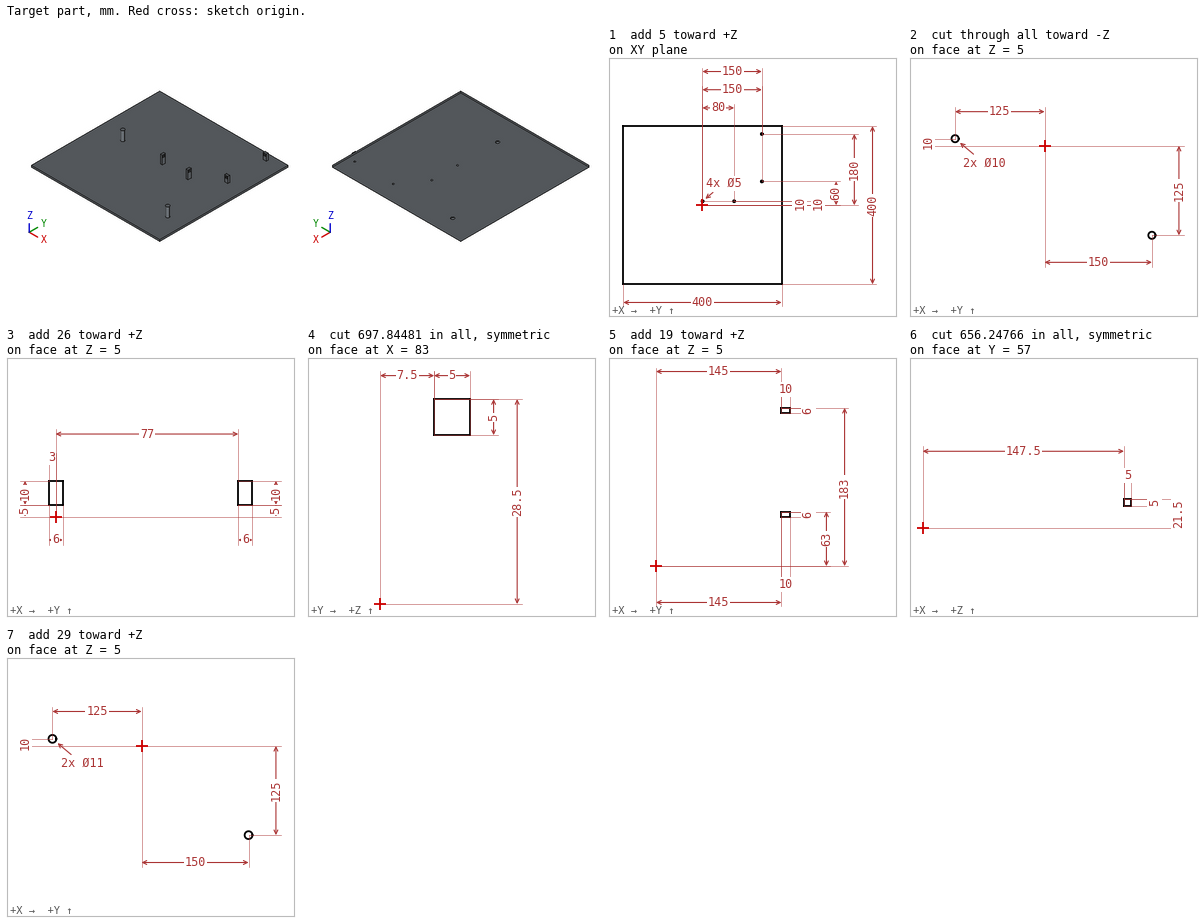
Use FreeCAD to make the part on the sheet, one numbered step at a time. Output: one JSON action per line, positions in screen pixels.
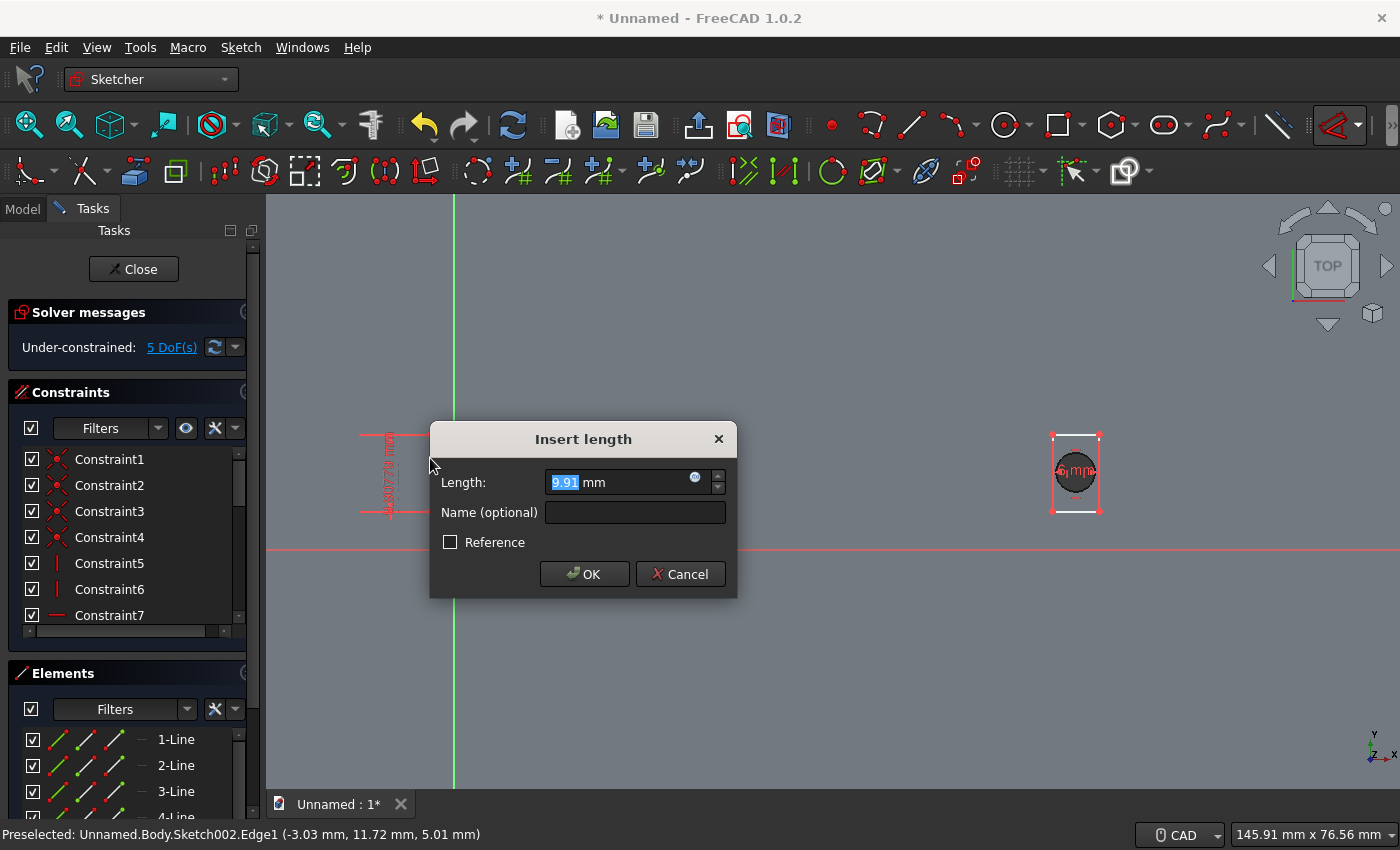
{"action": "type", "text": "10"}
{"action": "key", "text": "Return"}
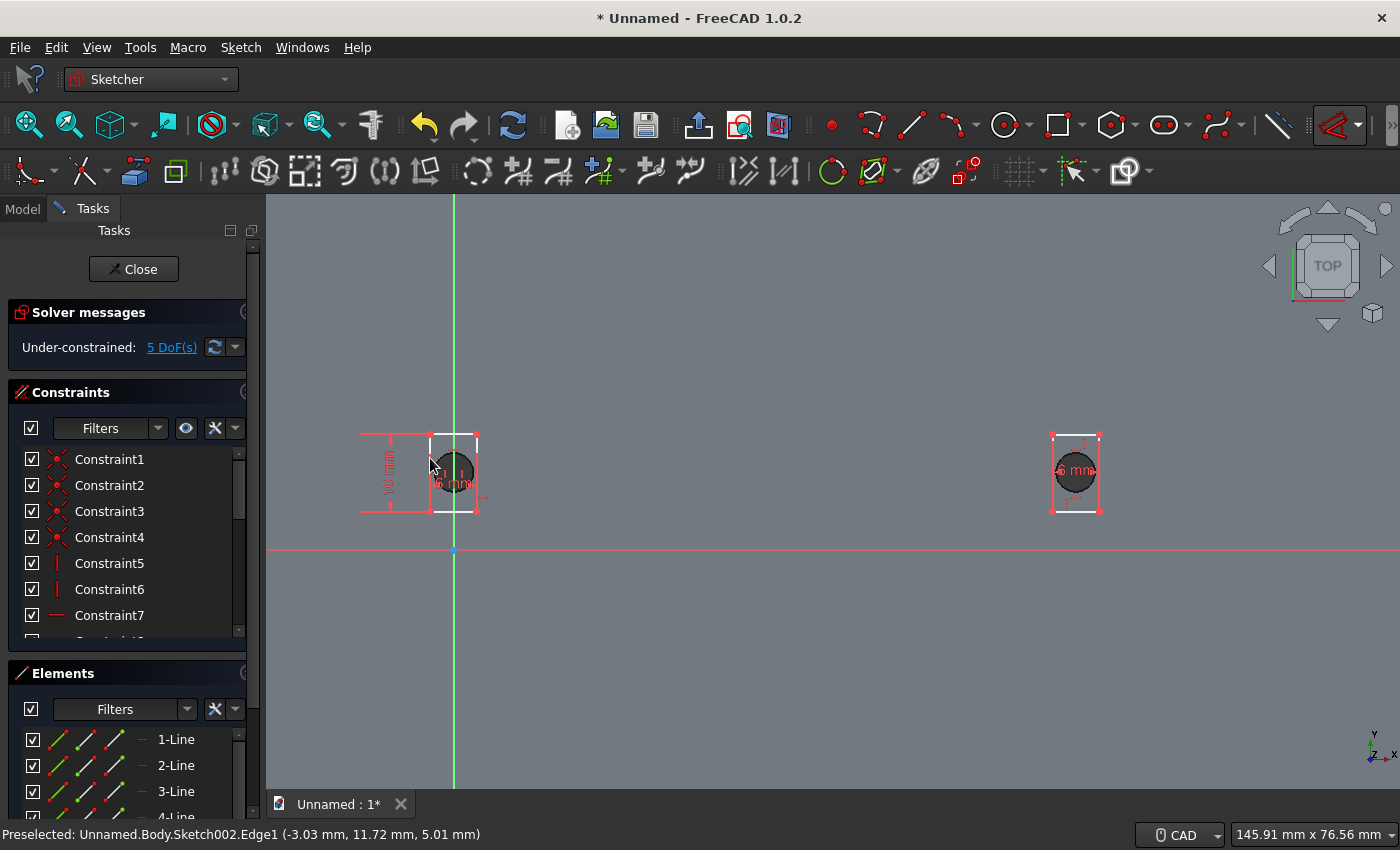
{"action": "left_click", "coordinate": [1053, 458]}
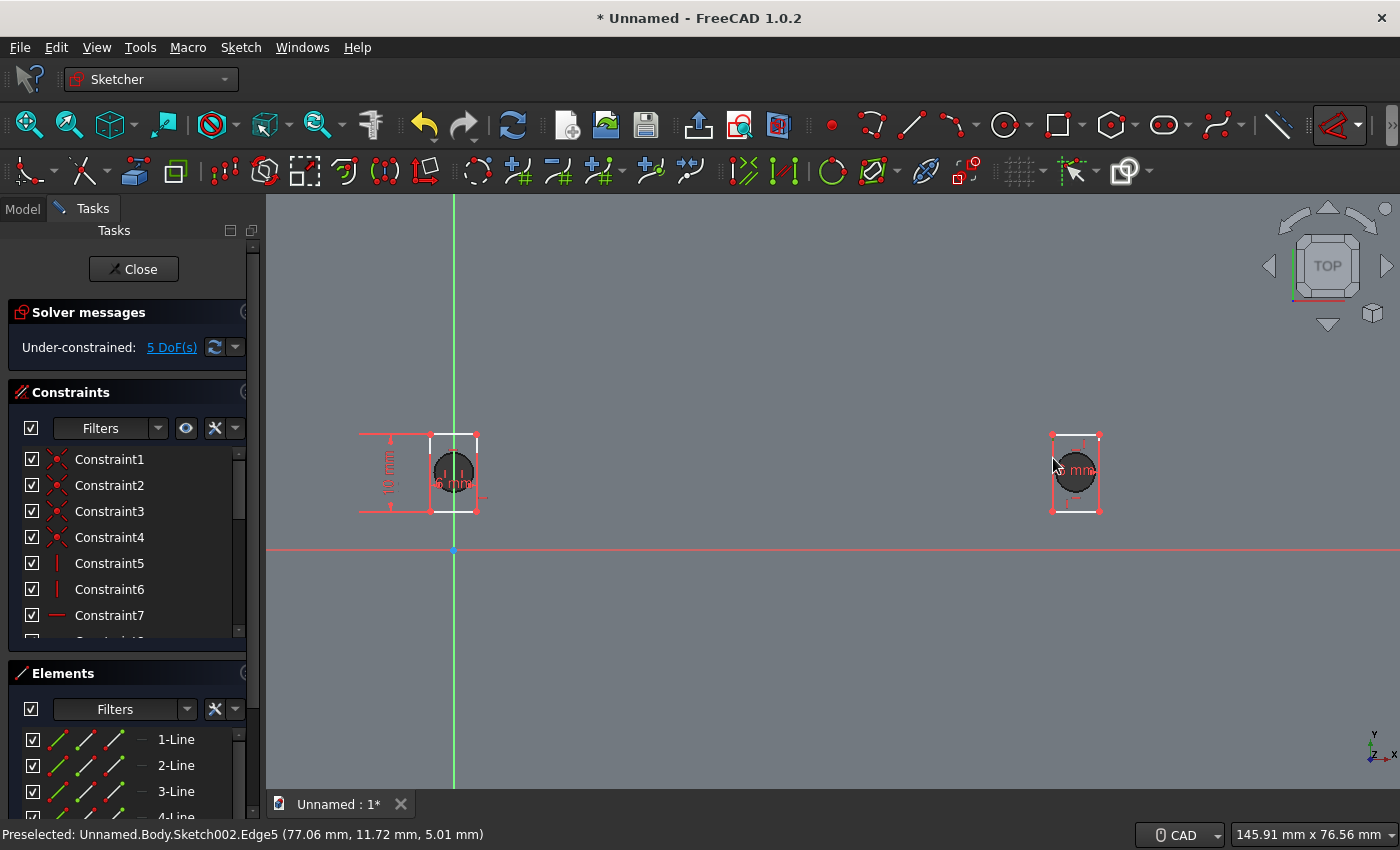
{"action": "key", "text": "i"}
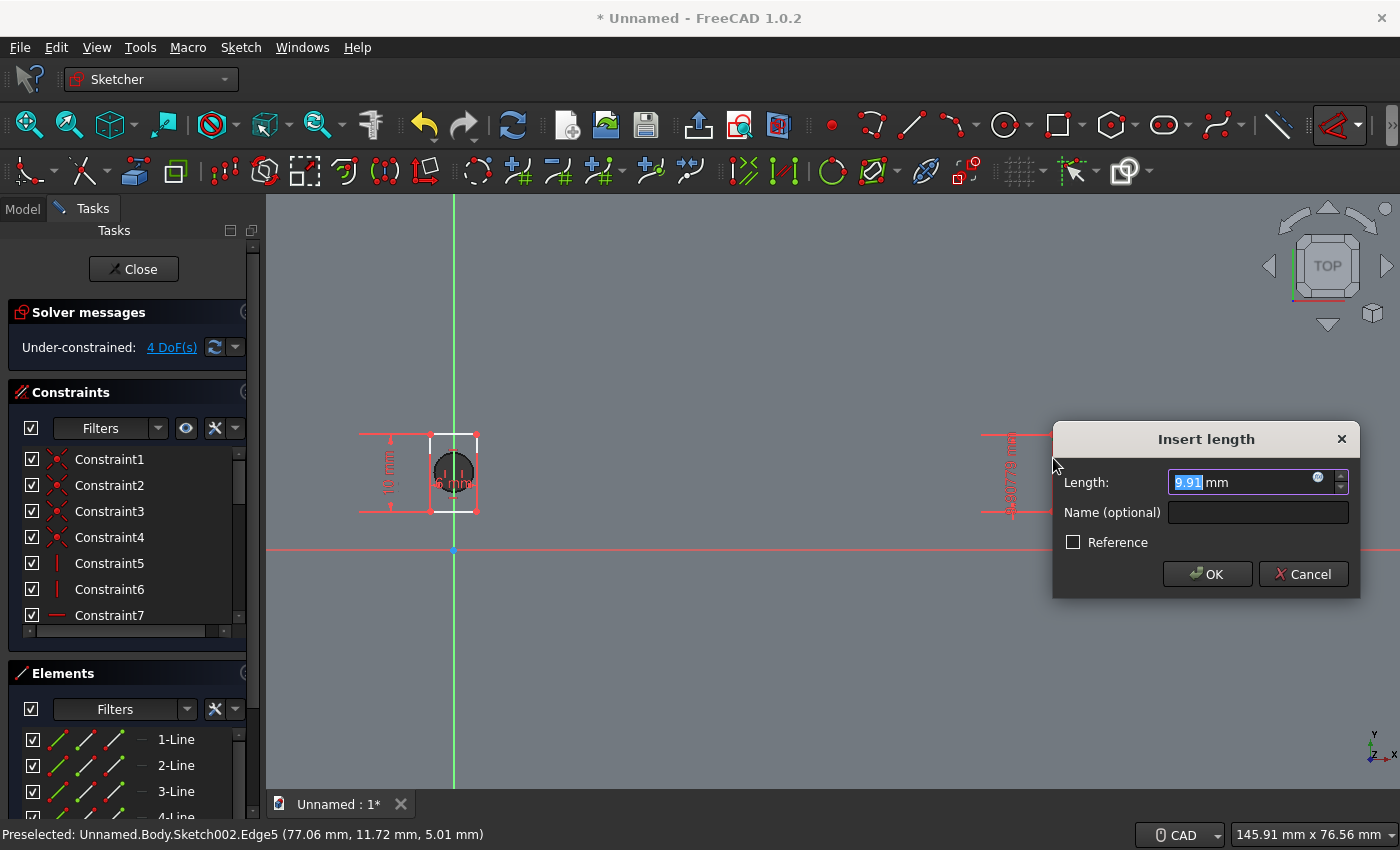
{"action": "type", "text": "10"}
{"action": "key", "text": "Return"}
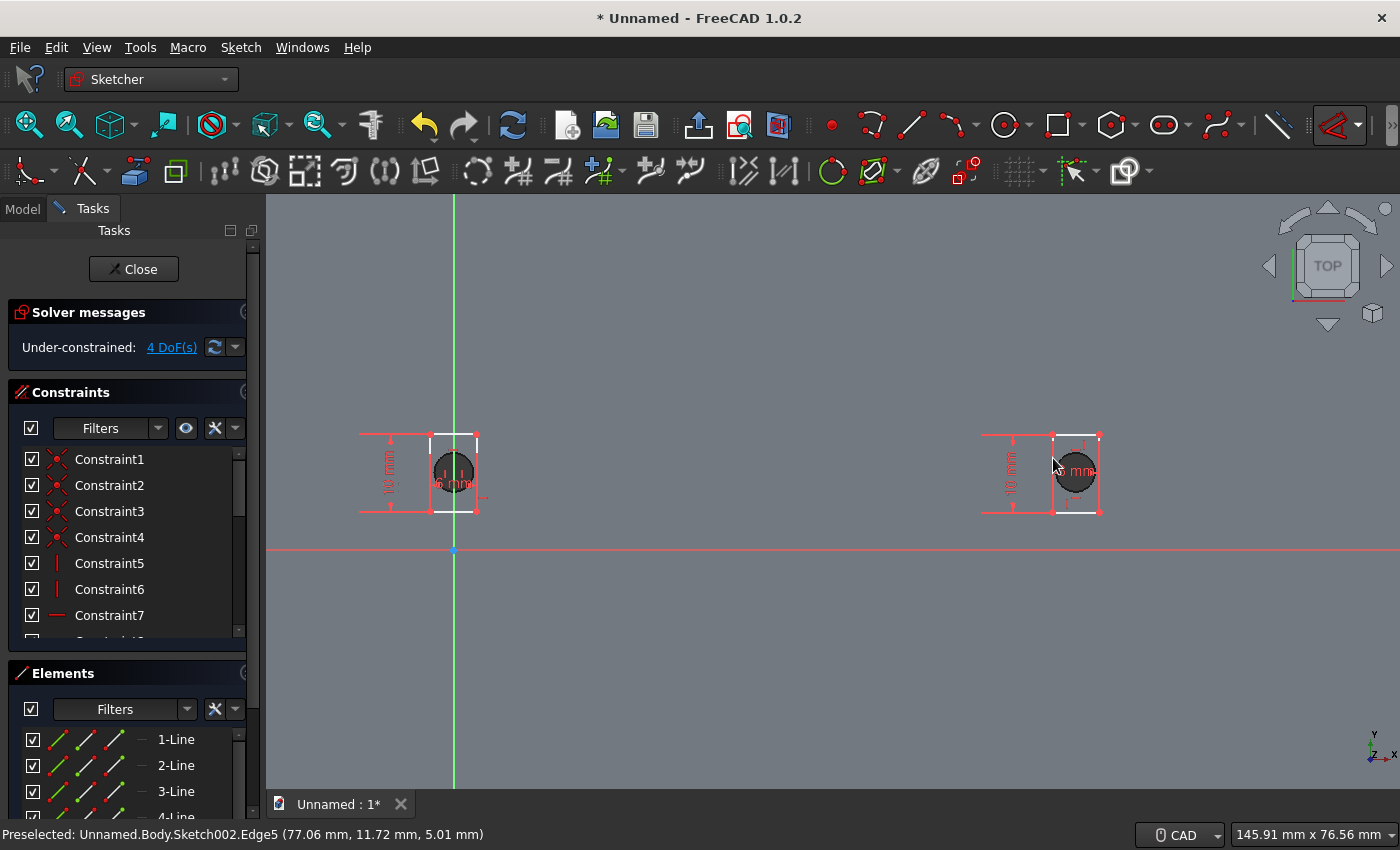
{"action": "scroll", "coordinate": [430, 434], "scroll_direction": "up", "scroll_amount": 3}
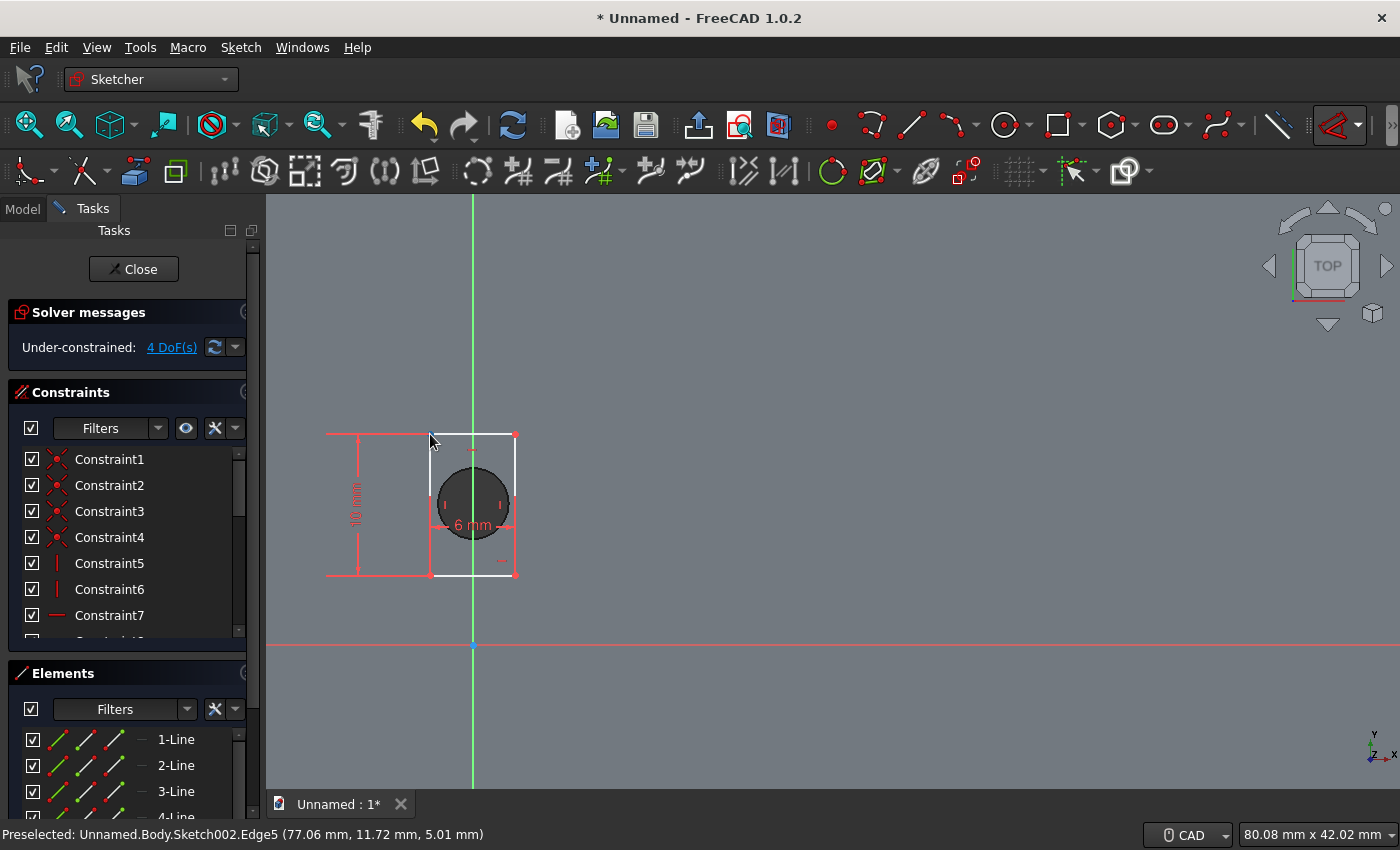
{"action": "left_click", "coordinate": [430, 434]}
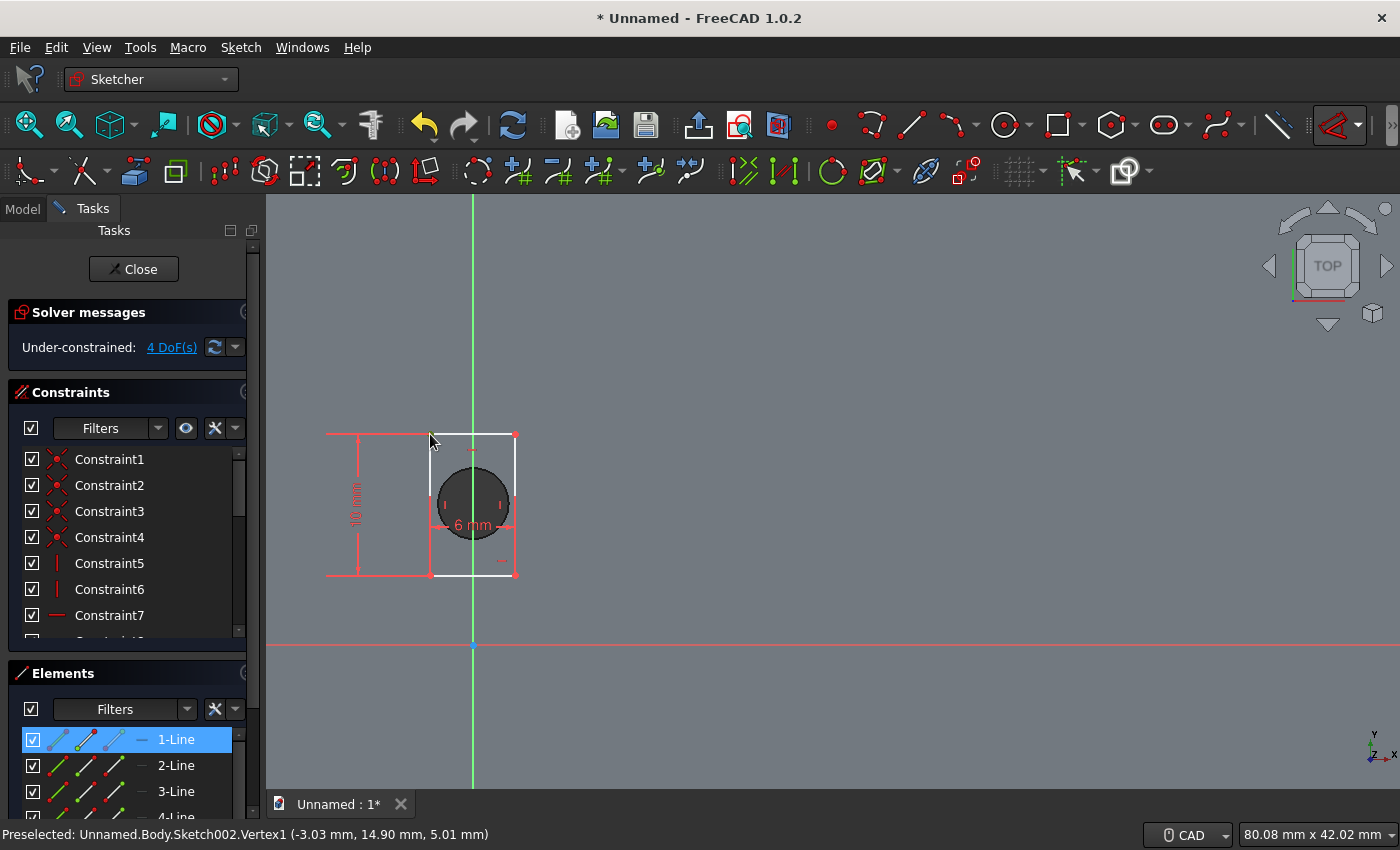
{"action": "key", "text": "l"}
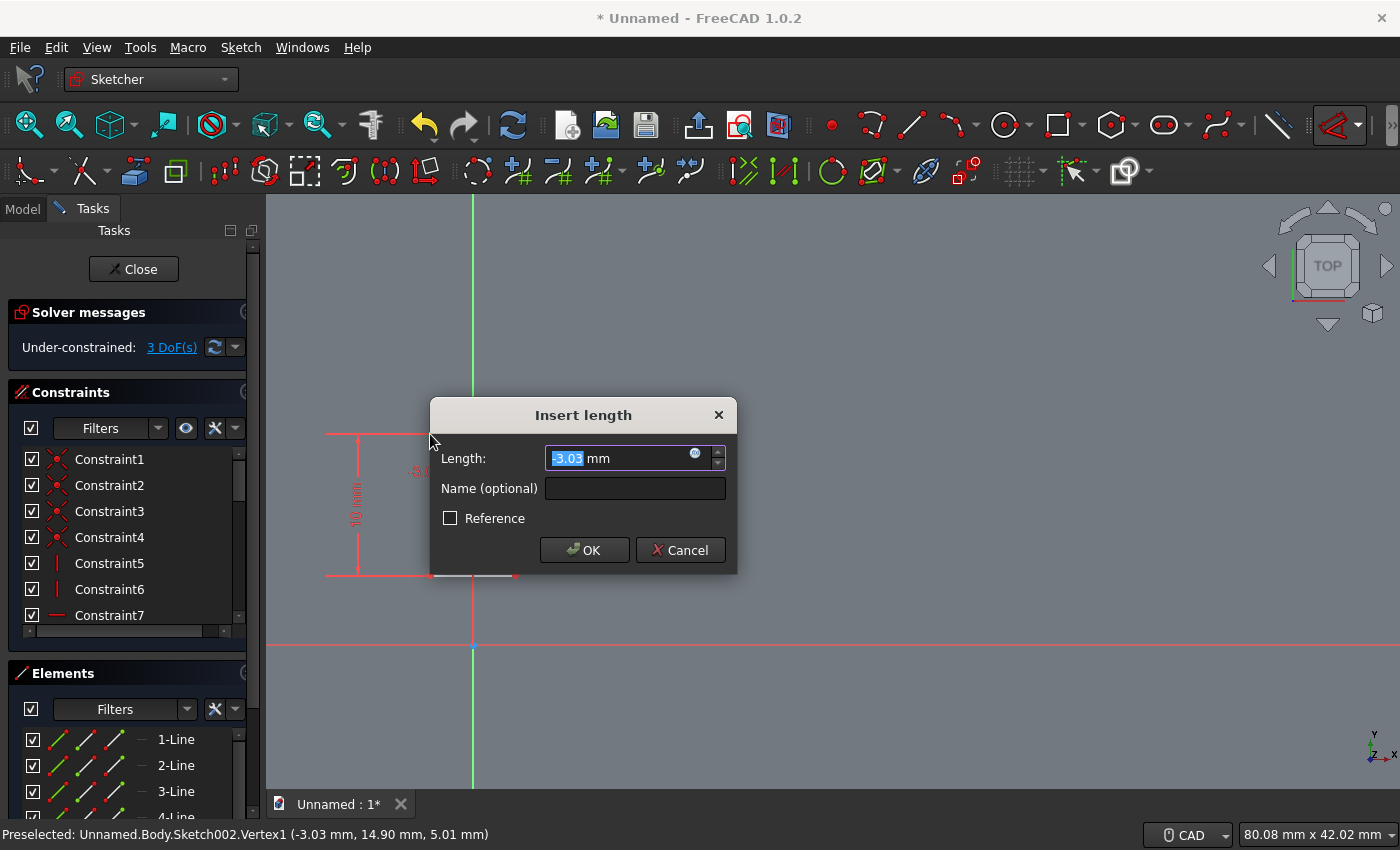
{"action": "type", "text": "-3"}
{"action": "key", "text": "Return"}